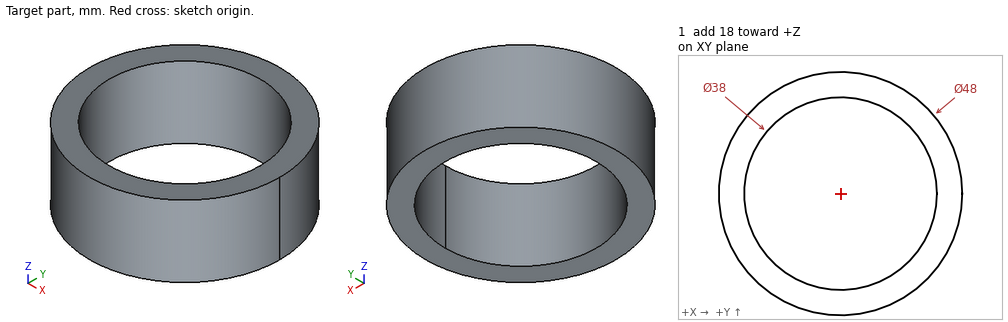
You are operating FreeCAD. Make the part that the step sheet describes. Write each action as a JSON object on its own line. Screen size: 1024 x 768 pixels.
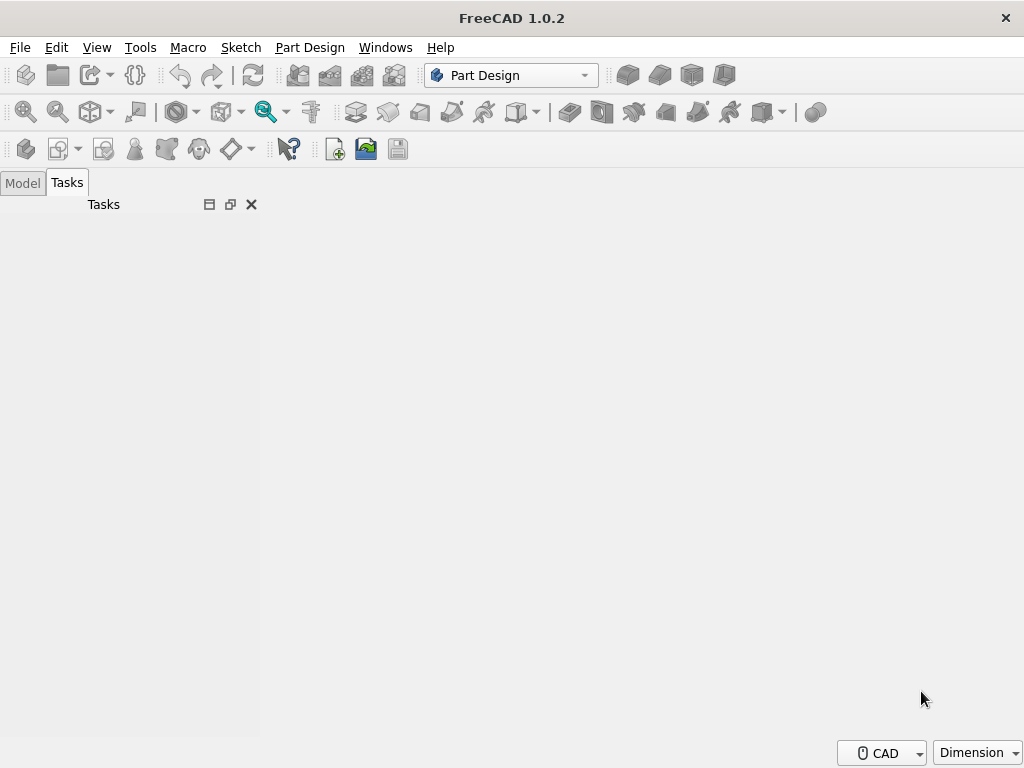
{"action": "left_click", "coordinate": [334, 150]}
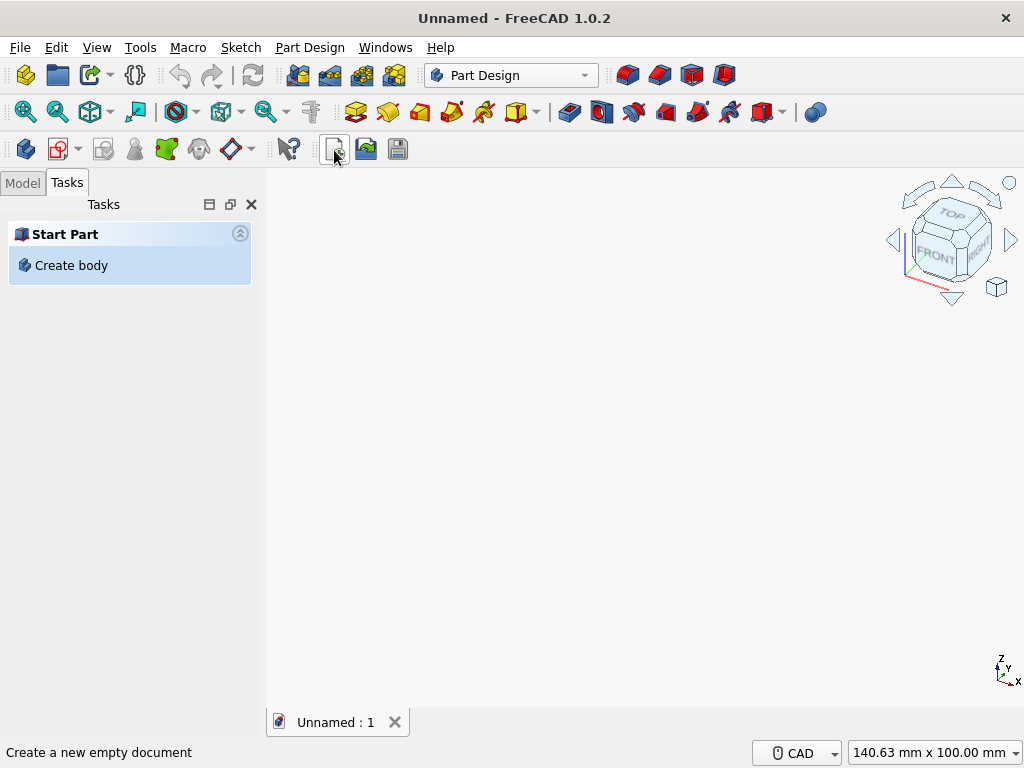
{"action": "left_click", "coordinate": [58, 150]}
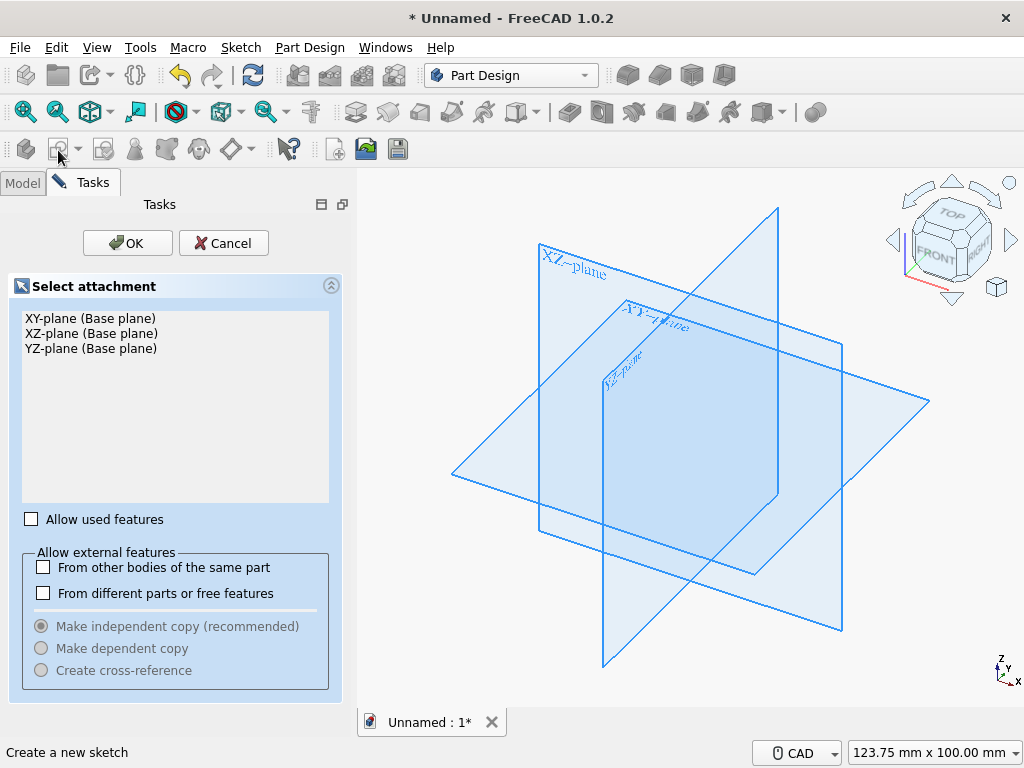
{"action": "left_click", "coordinate": [82, 318]}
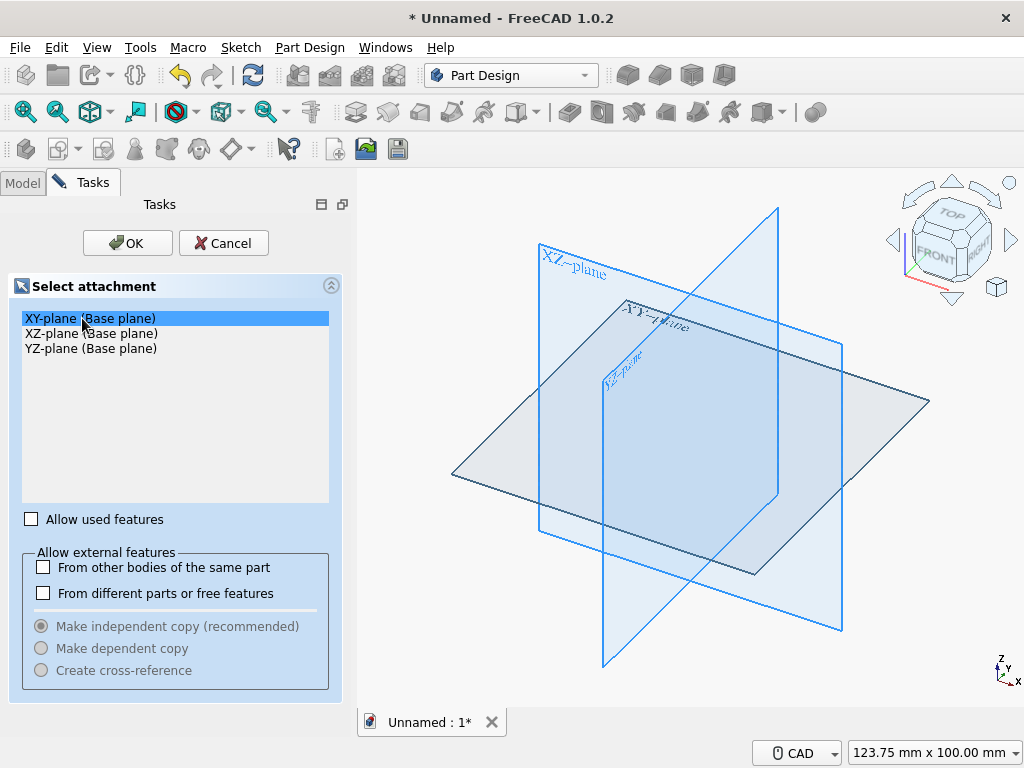
{"action": "left_click", "coordinate": [128, 243]}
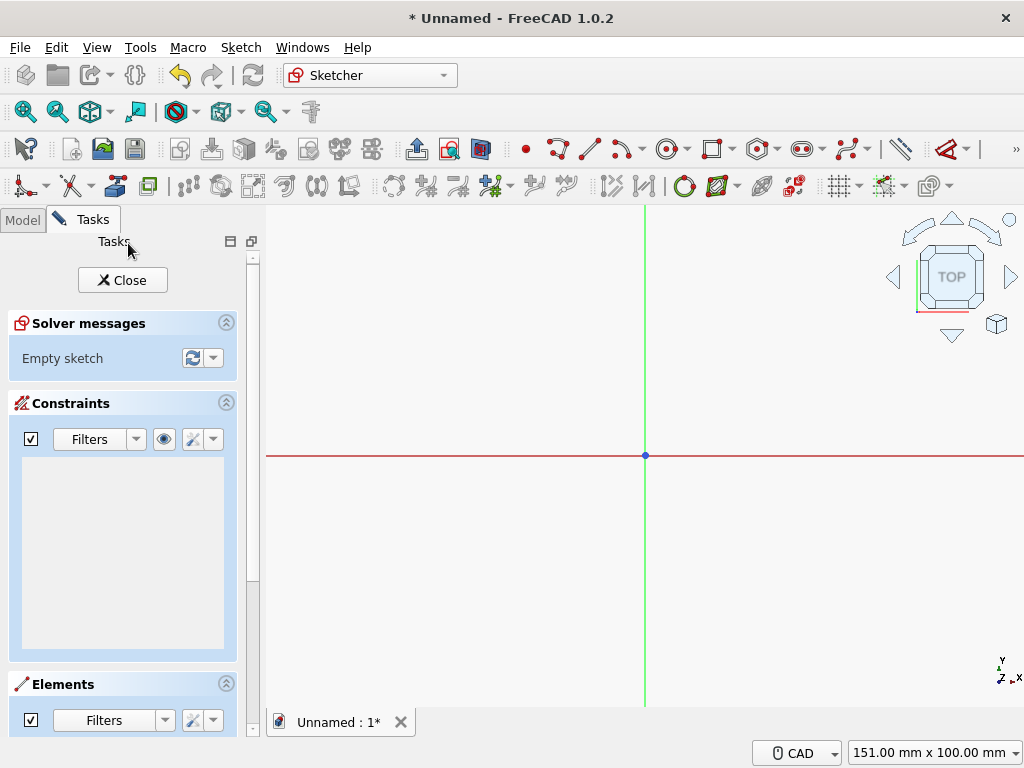
{"action": "left_click", "coordinate": [668, 150]}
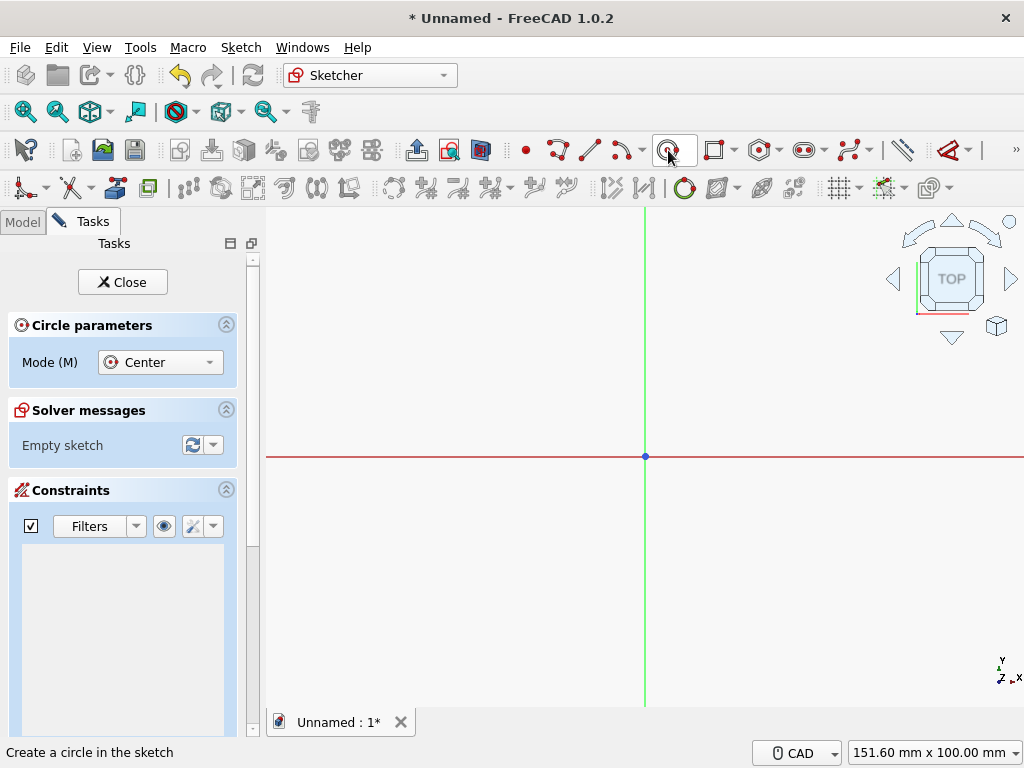
{"action": "left_click", "coordinate": [645, 457]}
{"action": "left_click", "coordinate": [730, 372]}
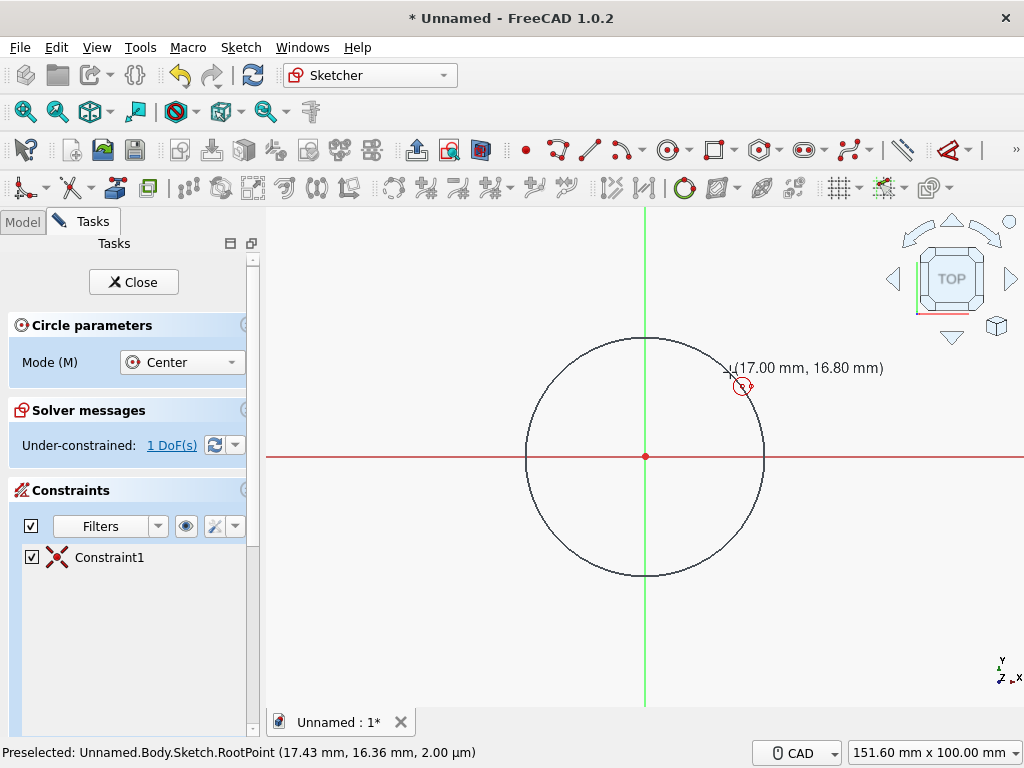
{"action": "left_click", "coordinate": [645, 457]}
{"action": "left_click", "coordinate": [712, 390]}
{"action": "key", "text": "Escape"}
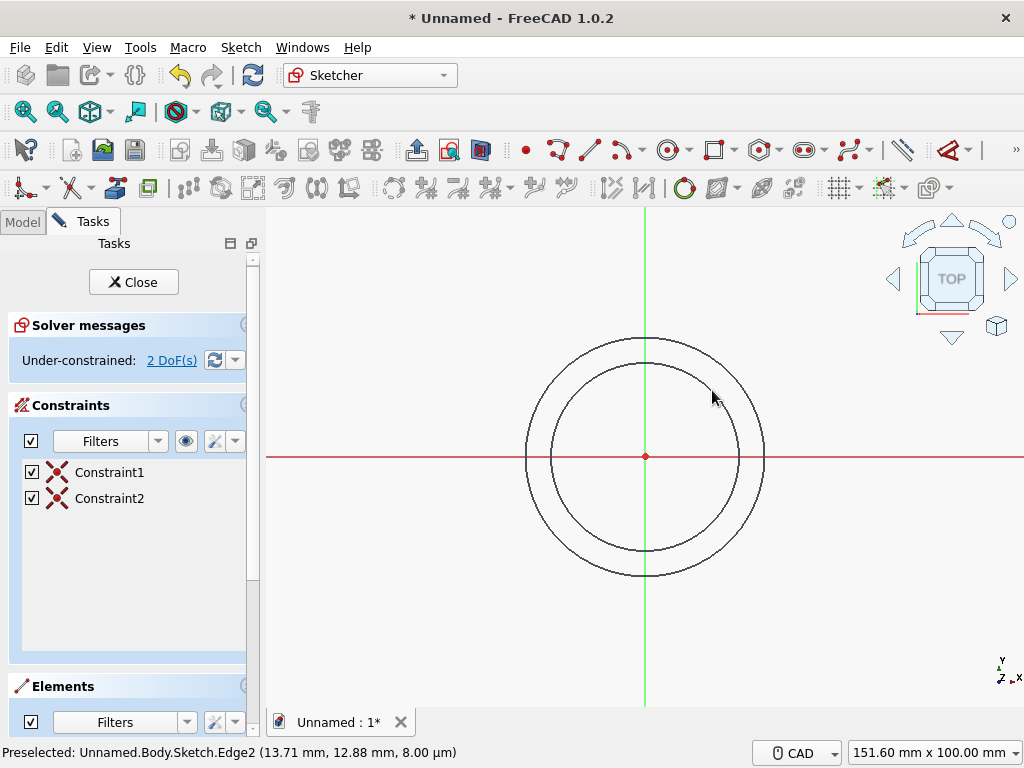
{"action": "left_click", "coordinate": [948, 150]}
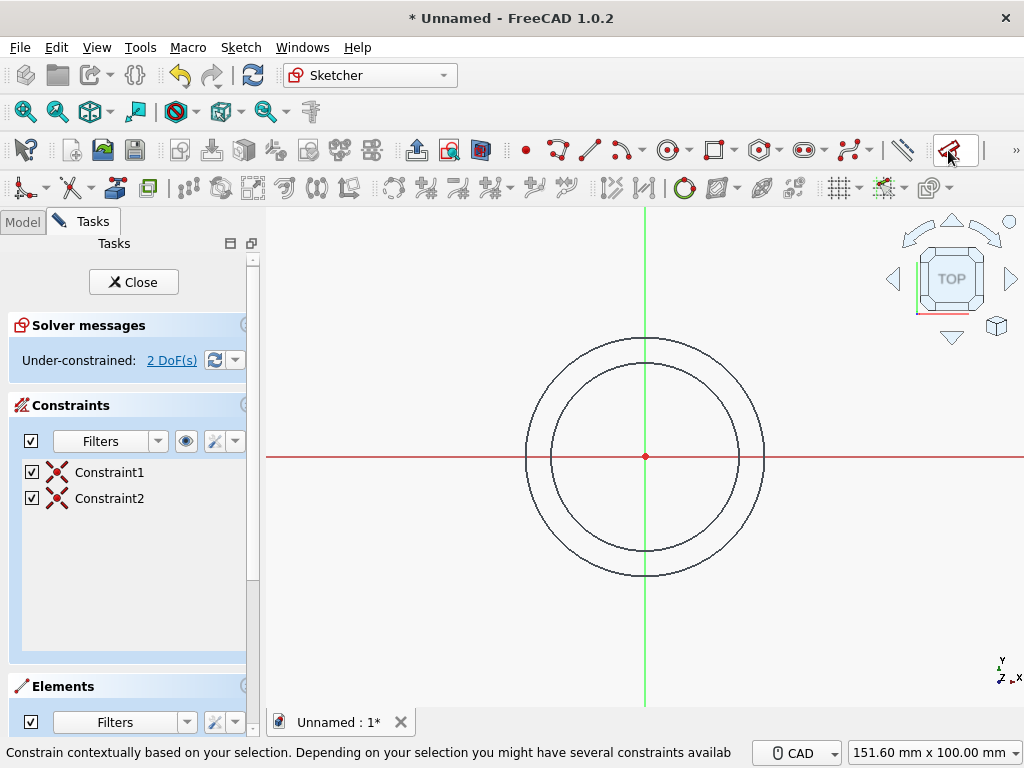
{"action": "left_click", "coordinate": [729, 372]}
{"action": "left_click", "coordinate": [751, 349]}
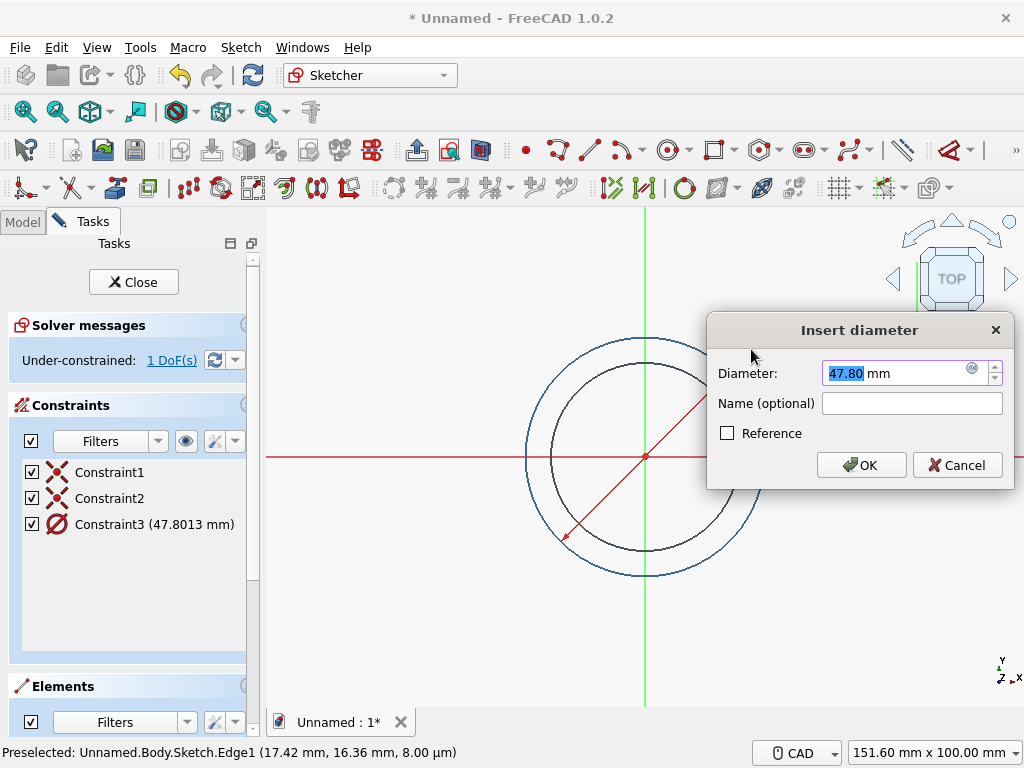
{"action": "type", "text": "48"}
{"action": "key", "text": "Return"}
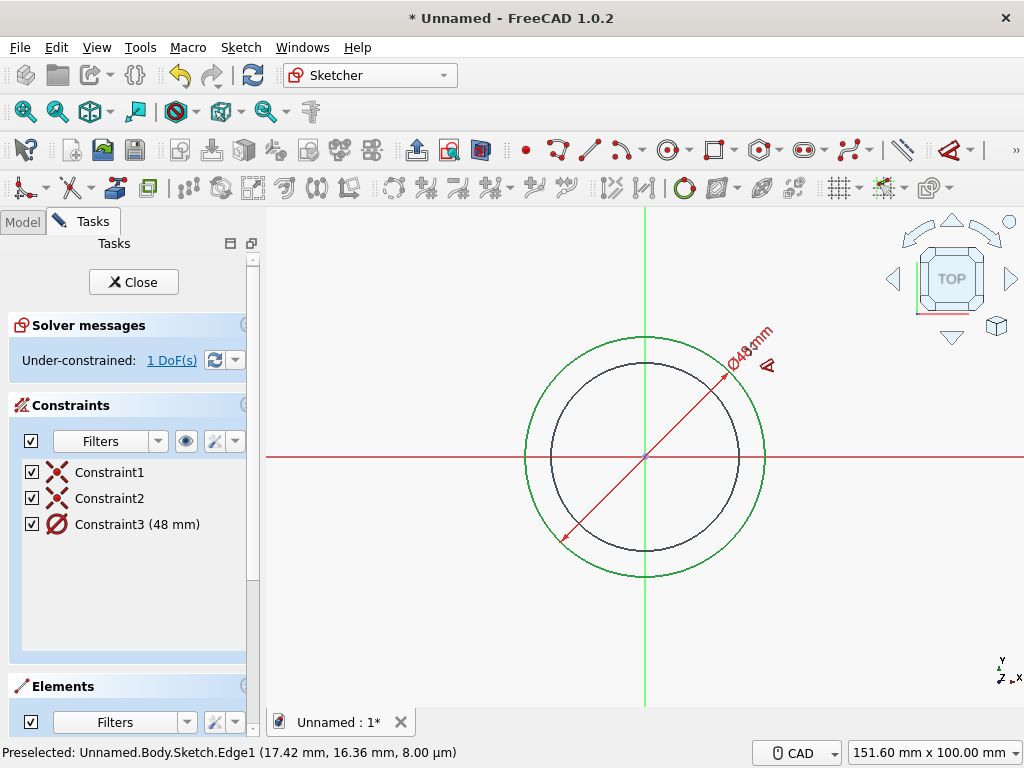
{"action": "left_click", "coordinate": [711, 390]}
{"action": "left_click", "coordinate": [788, 414]}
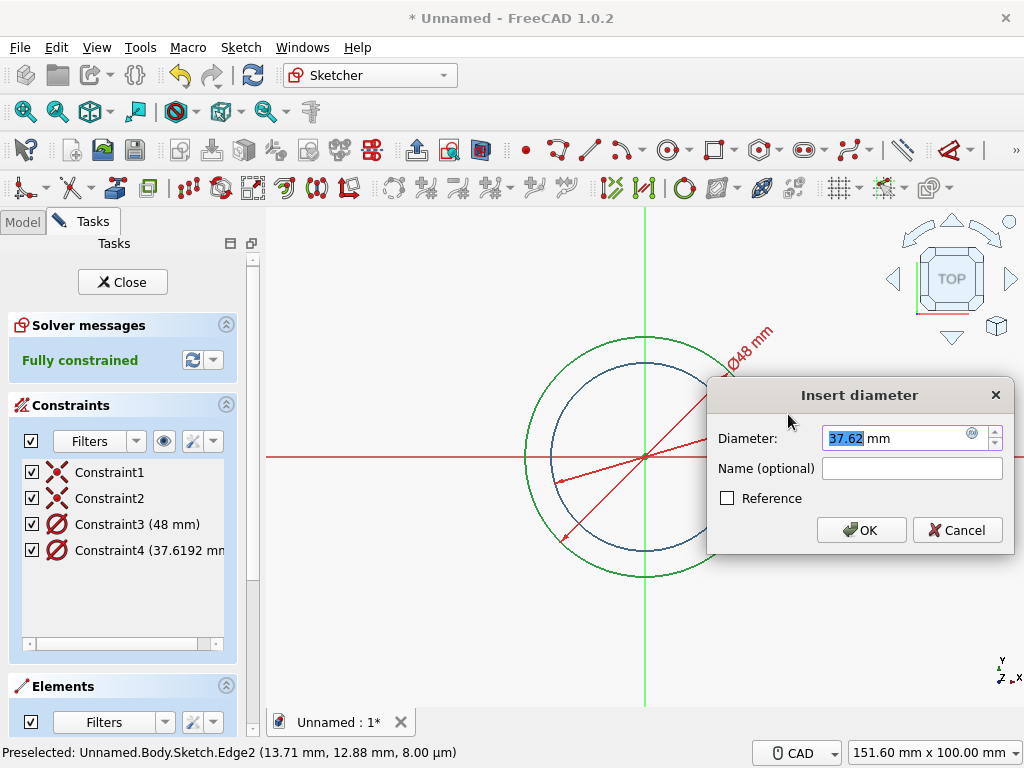
{"action": "type", "text": "38"}
{"action": "key", "text": "Return"}
{"action": "key", "text": "Escape"}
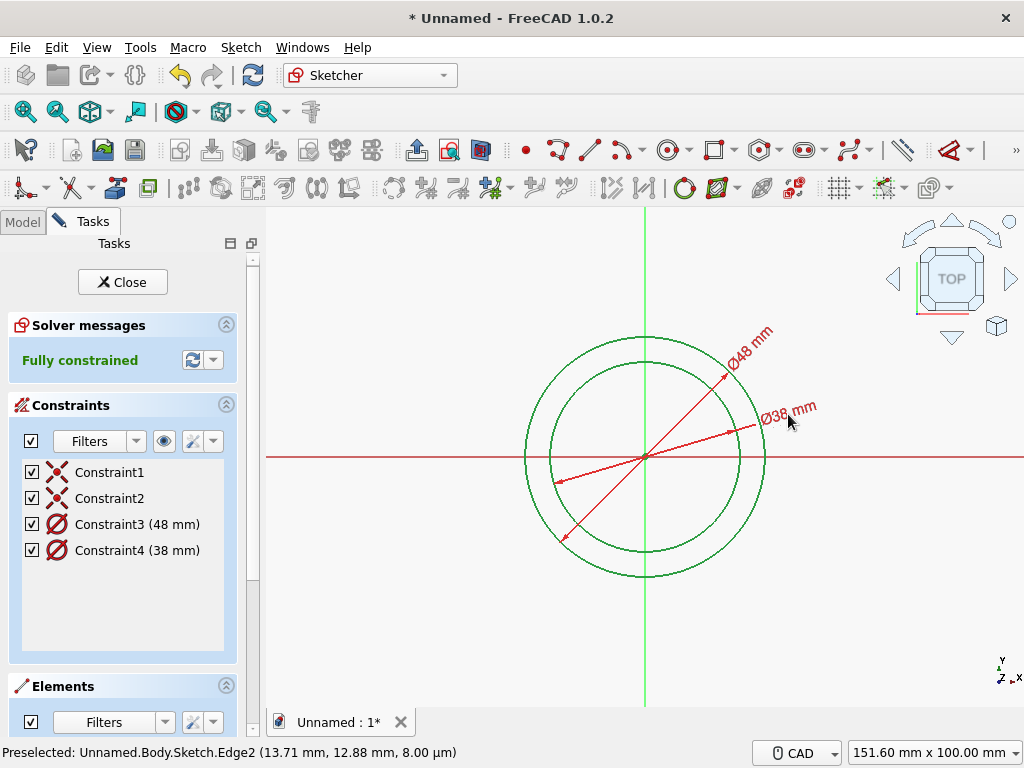
{"action": "left_click", "coordinate": [123, 282]}